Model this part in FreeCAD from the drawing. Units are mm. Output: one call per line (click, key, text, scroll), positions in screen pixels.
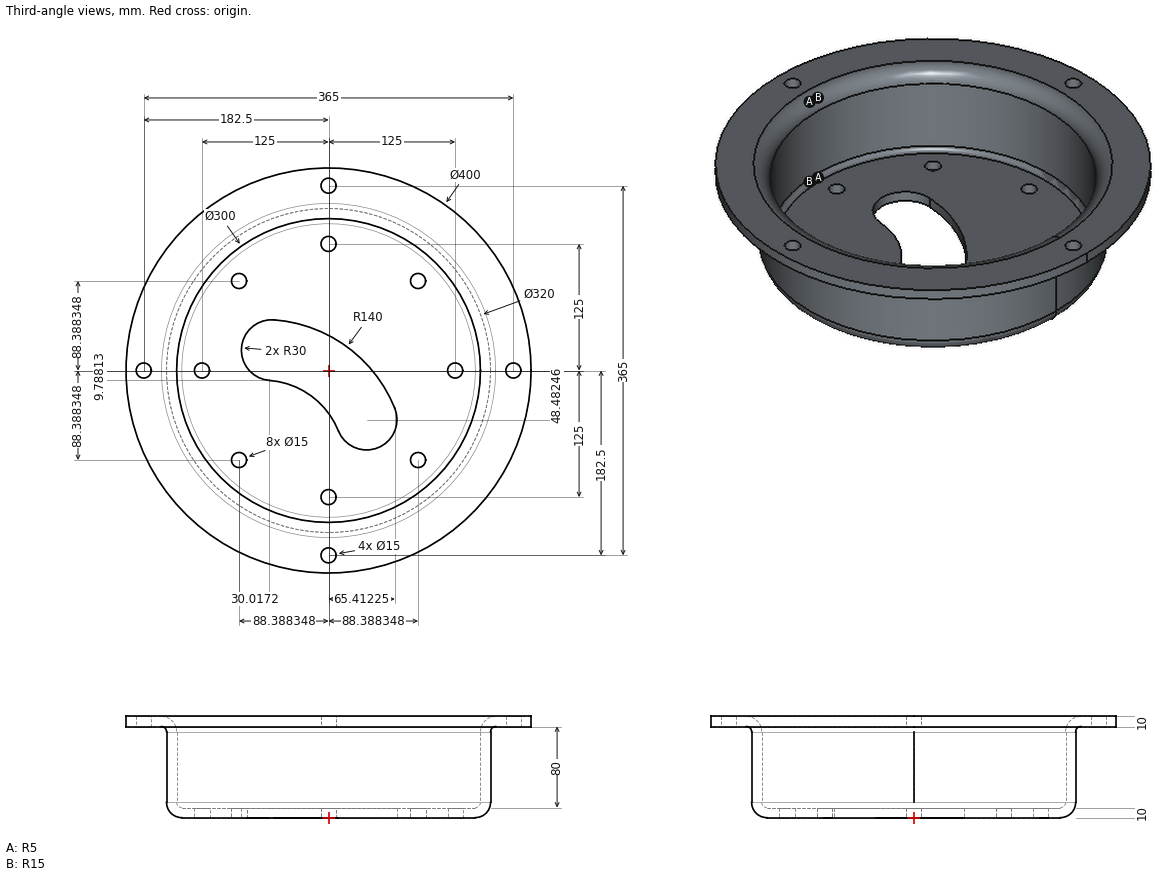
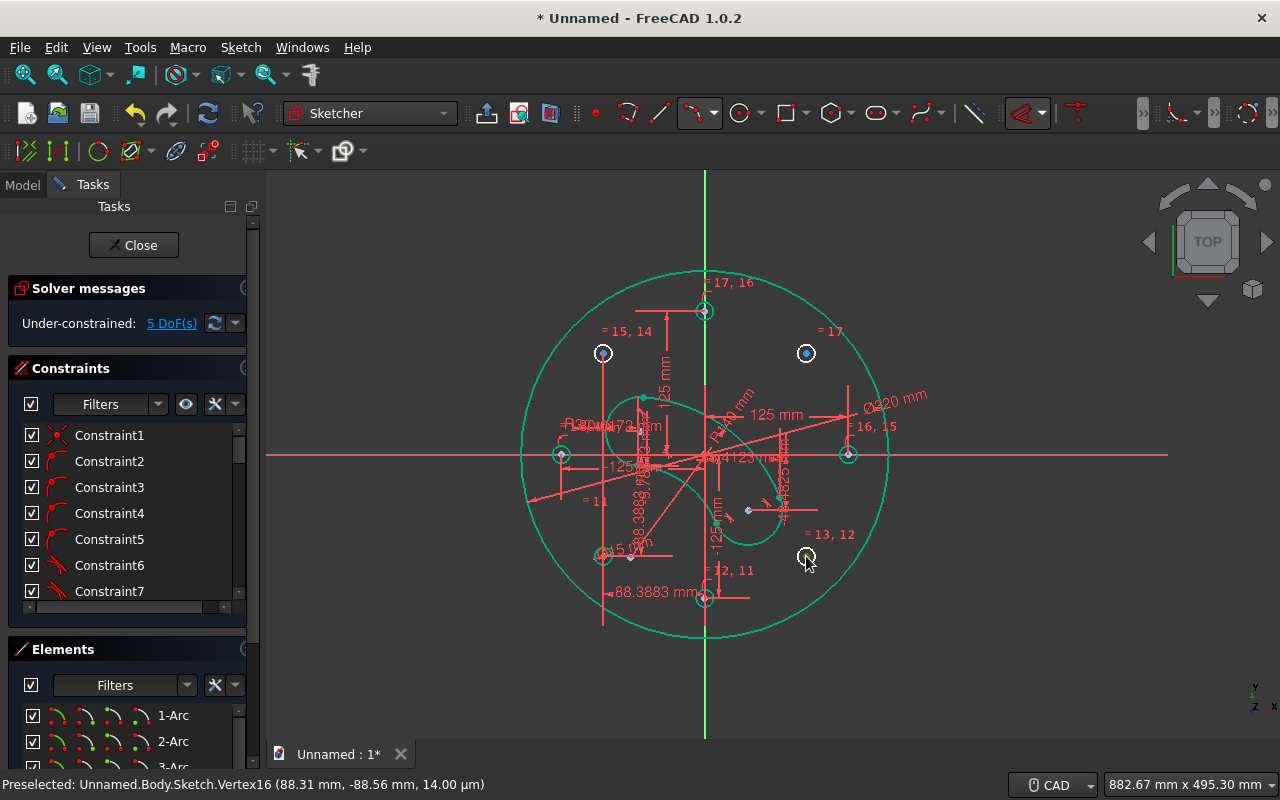
key(l)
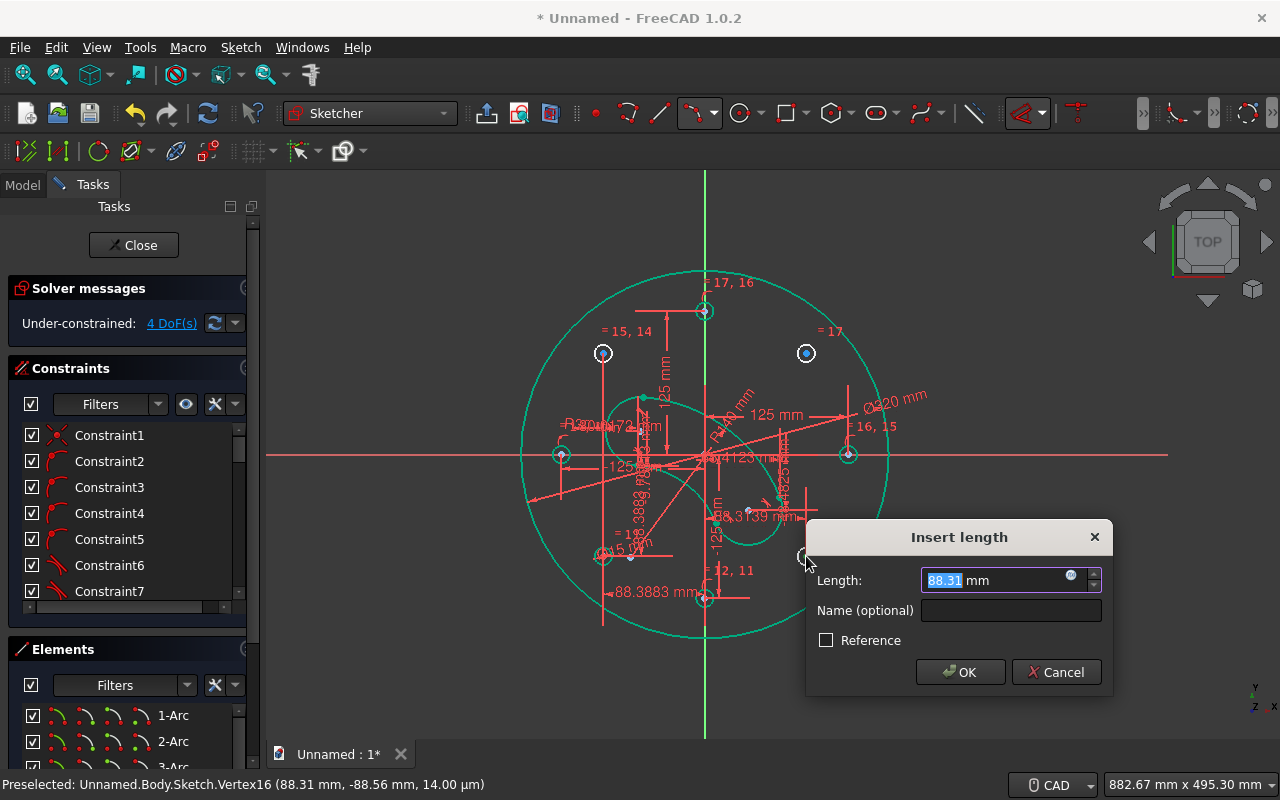
text(88.388348)
key(Return)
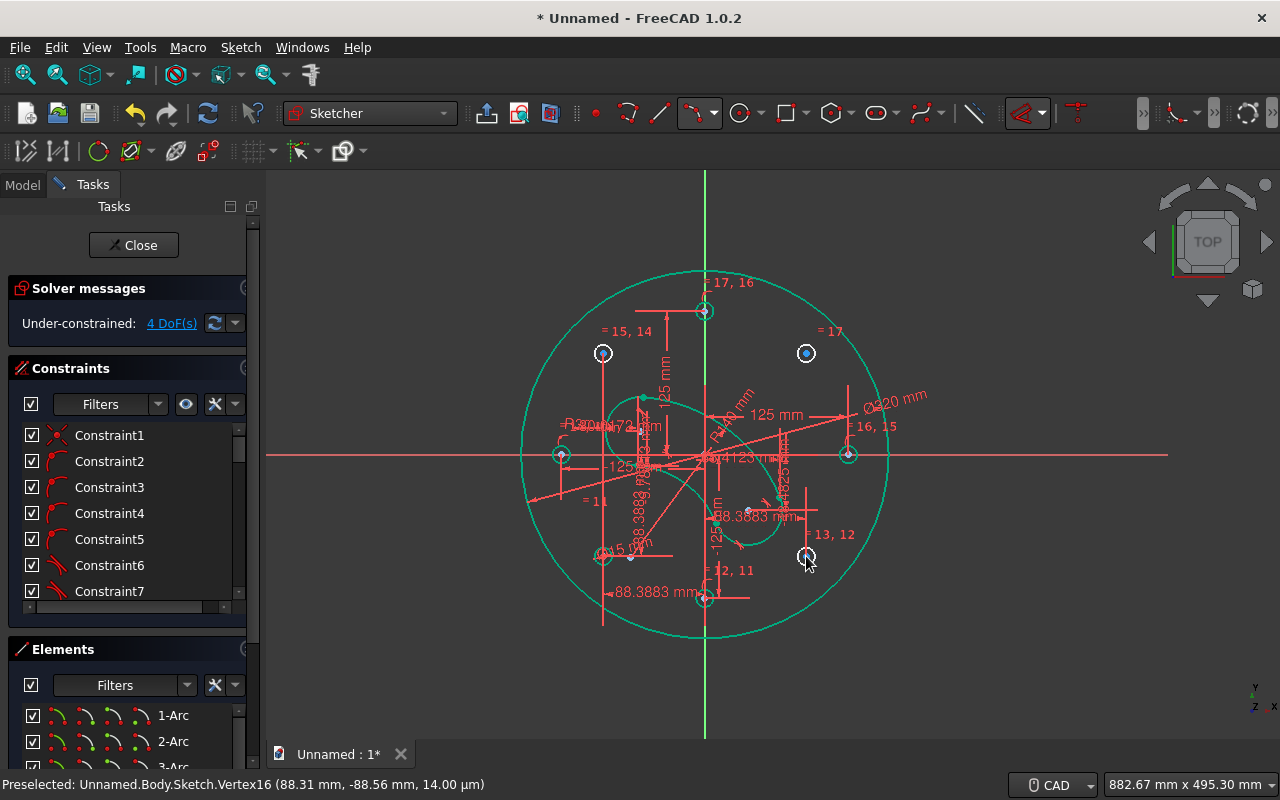
click(806, 556)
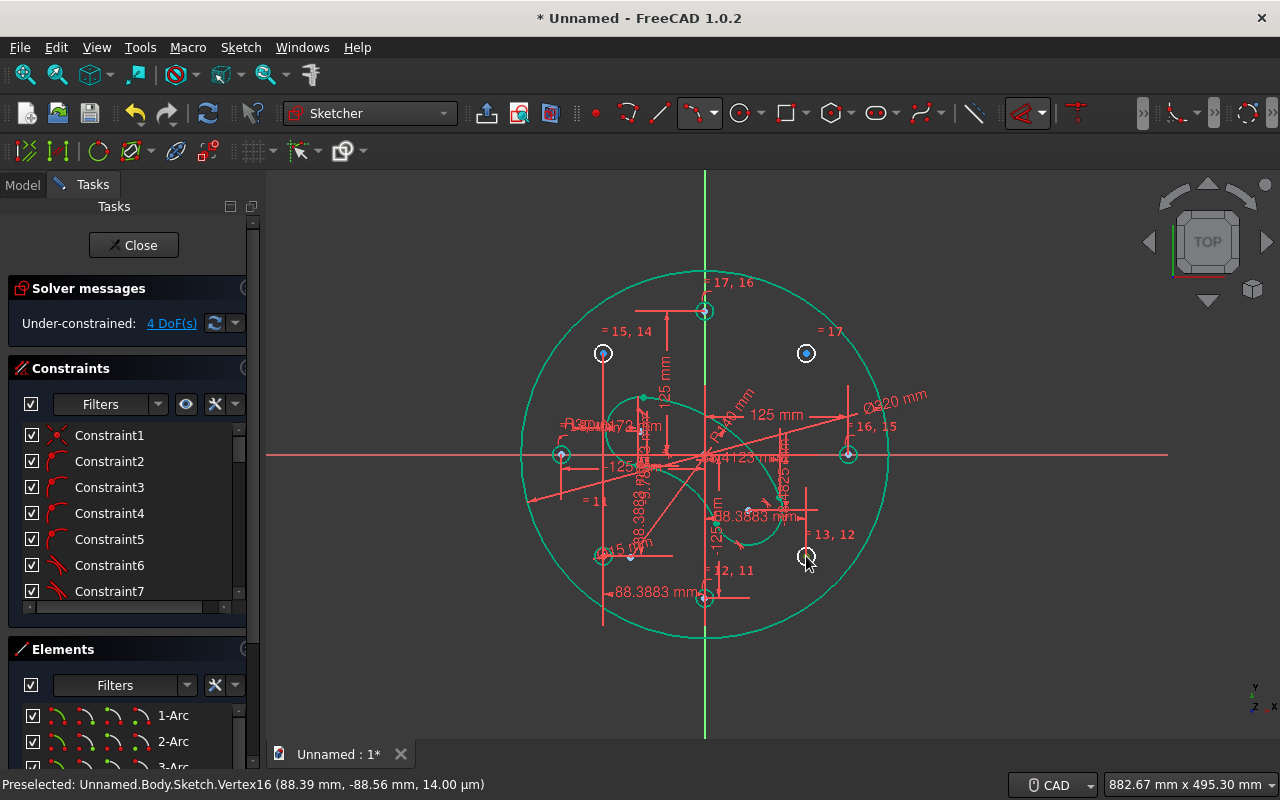
click(1044, 114)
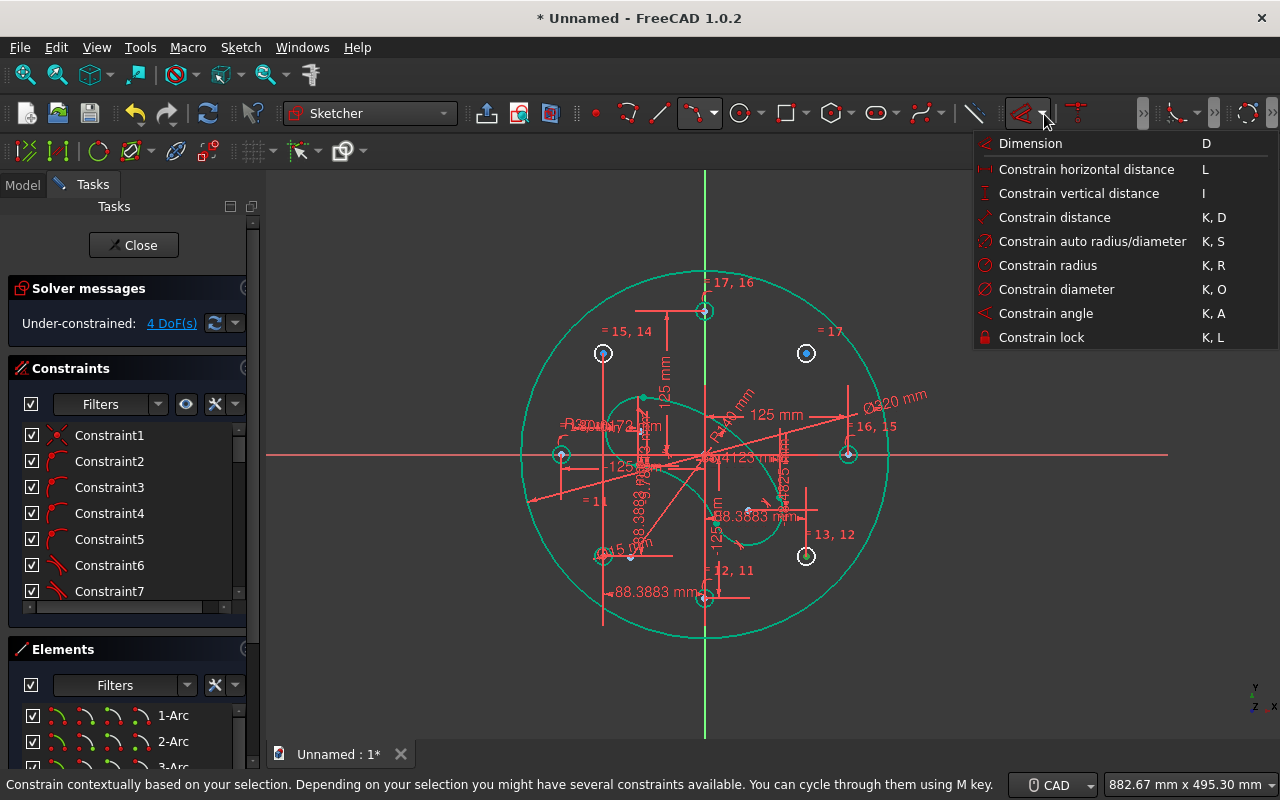
click(1126, 193)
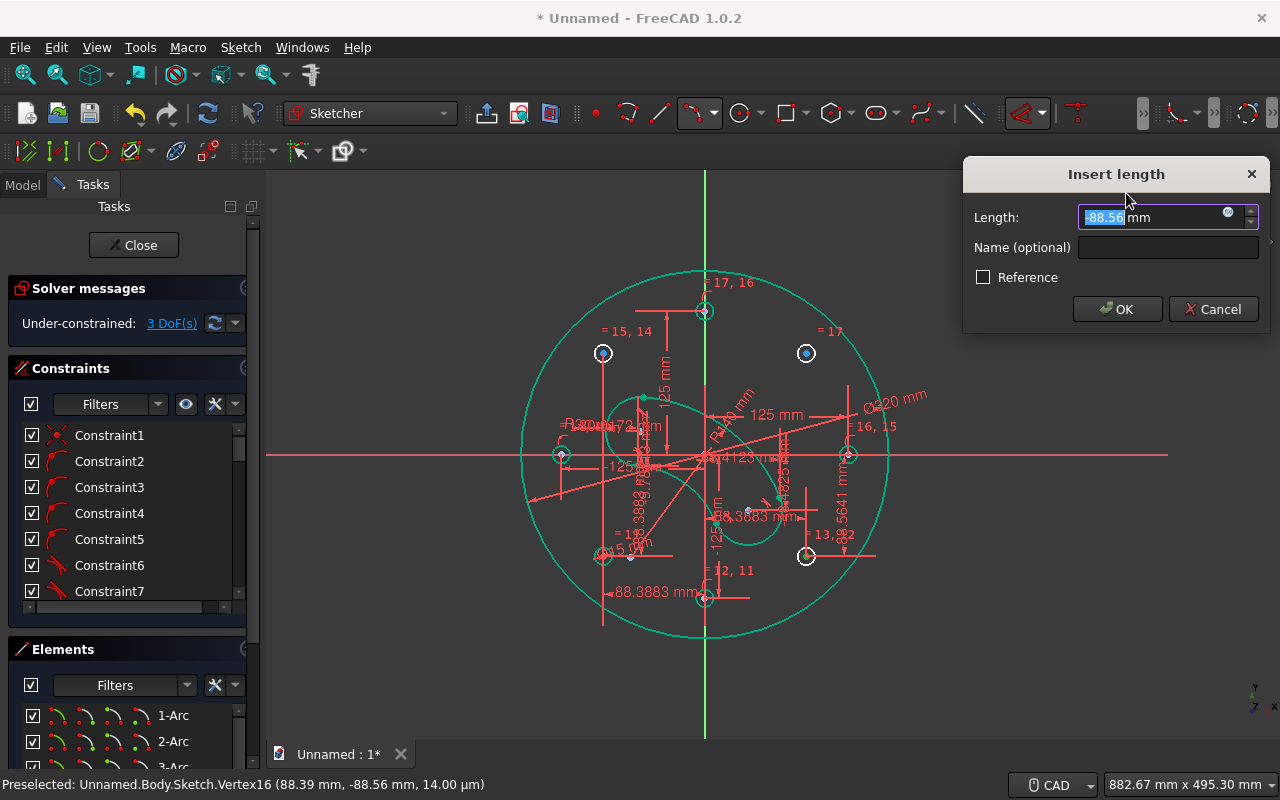
text(-88.388348)
key(Return)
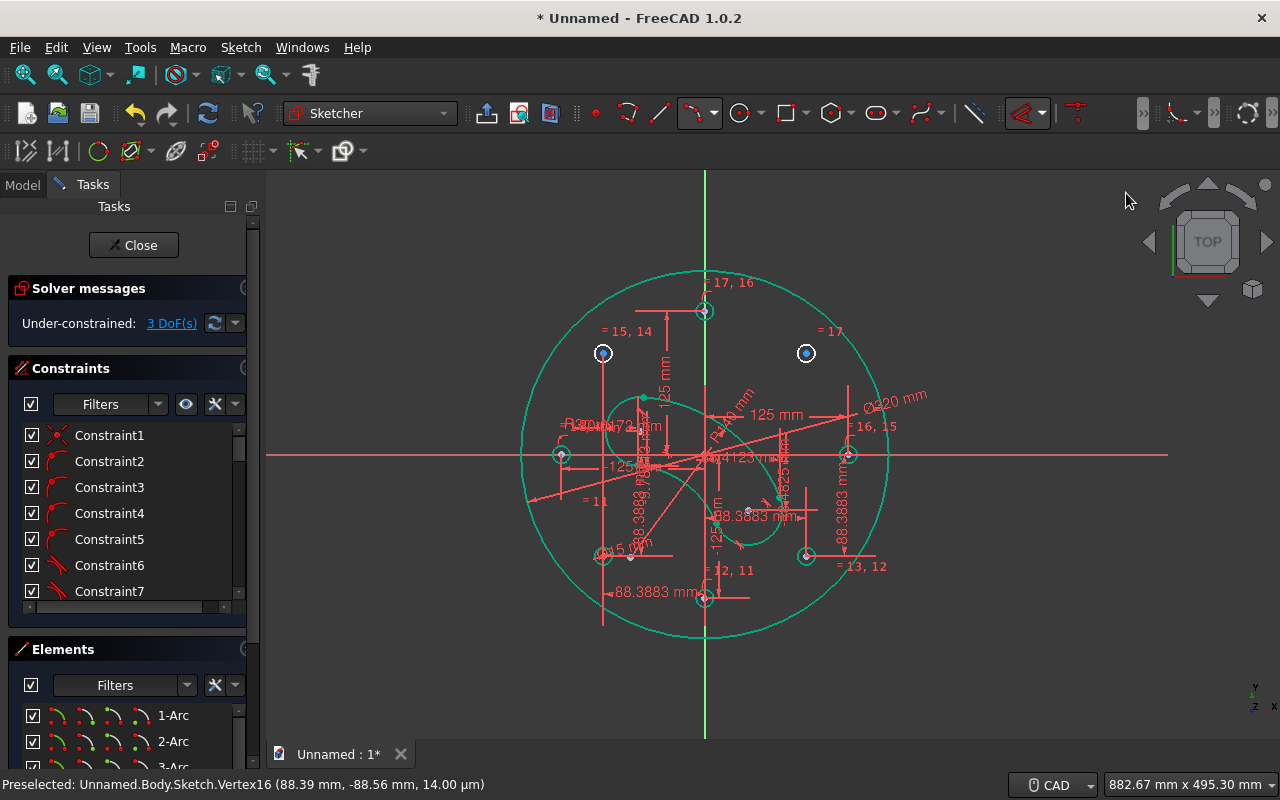
click(603, 353)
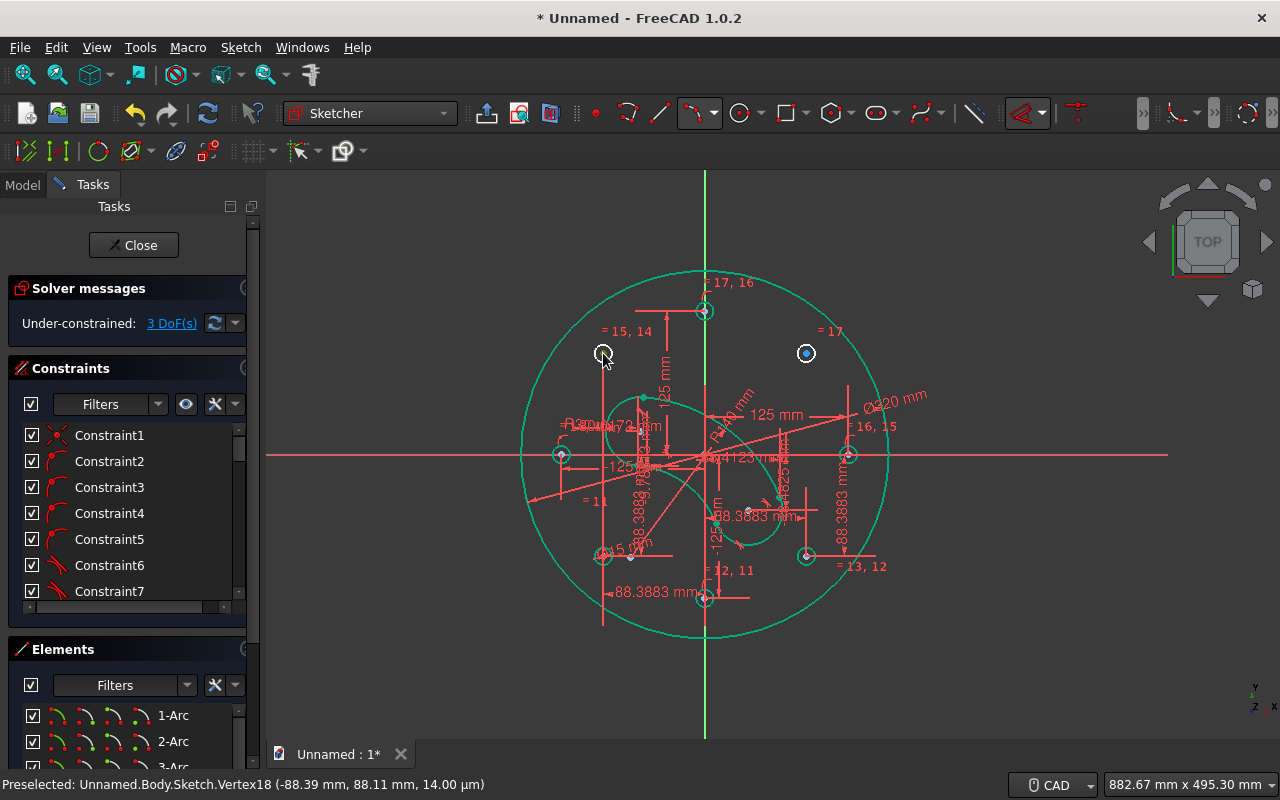
click(1044, 114)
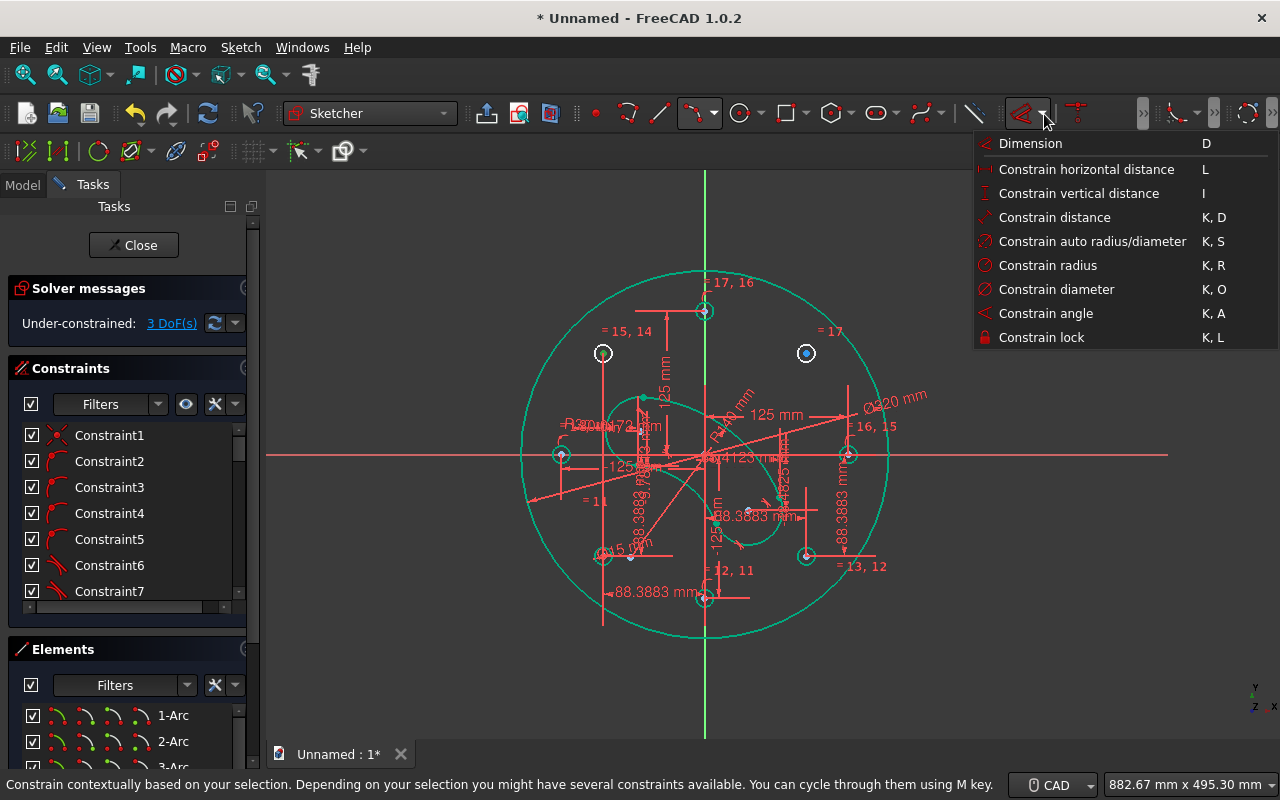
click(1126, 193)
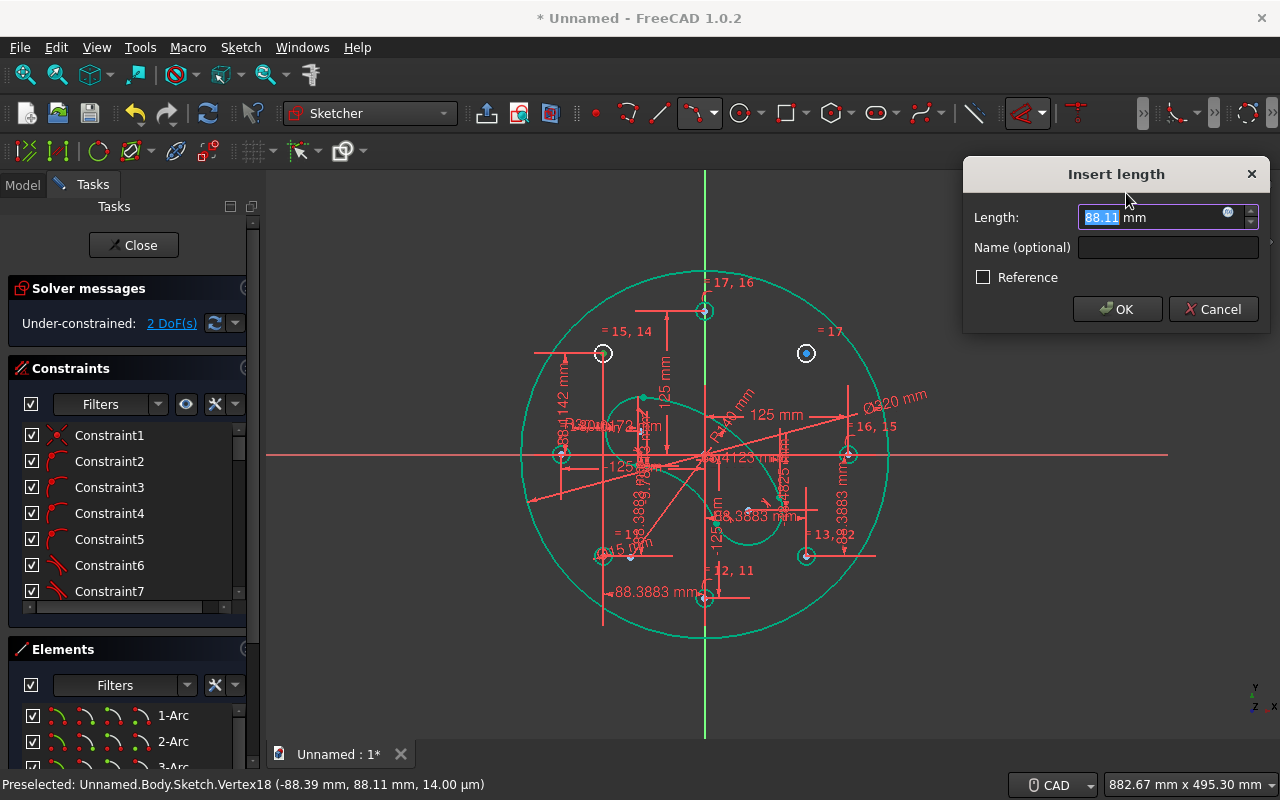
text(88.388348)
key(Return)